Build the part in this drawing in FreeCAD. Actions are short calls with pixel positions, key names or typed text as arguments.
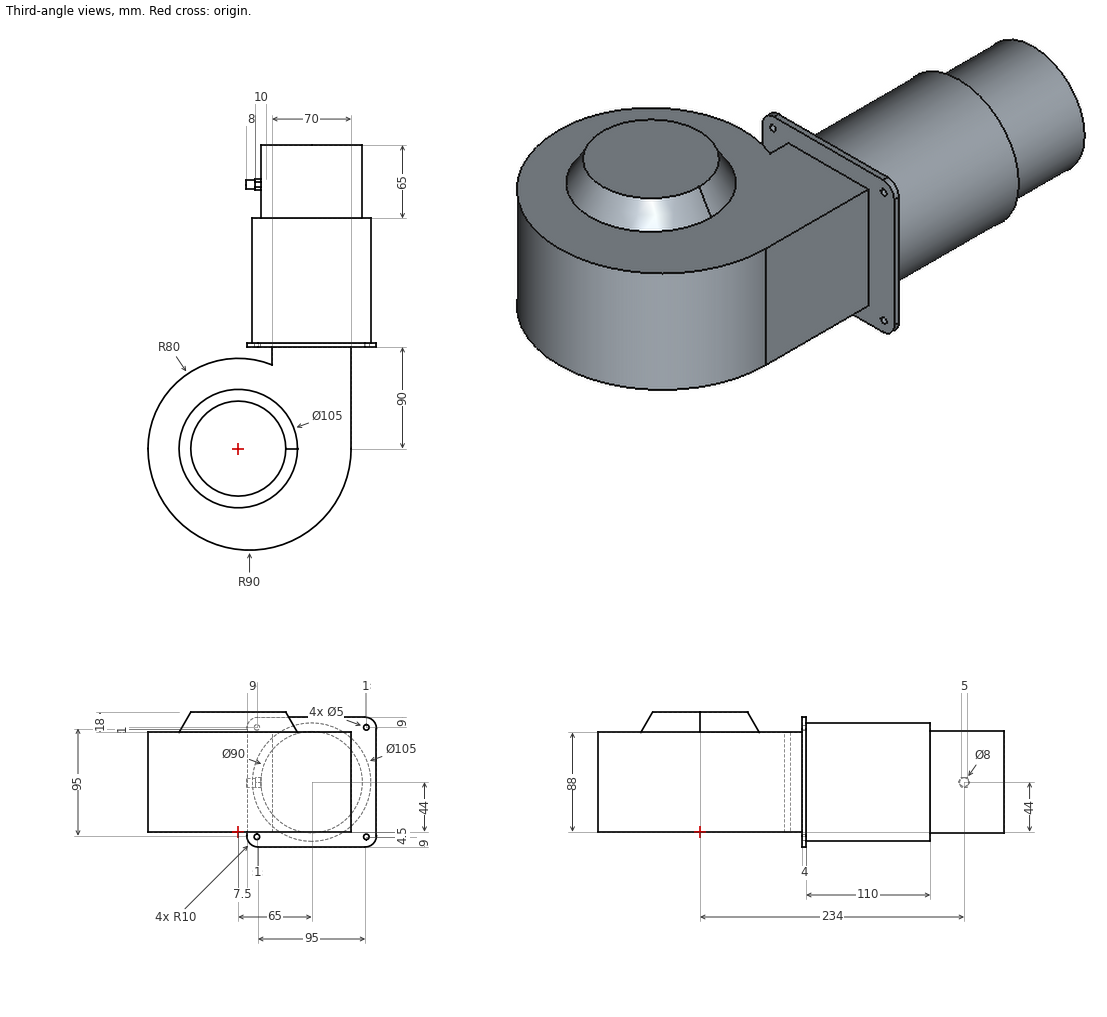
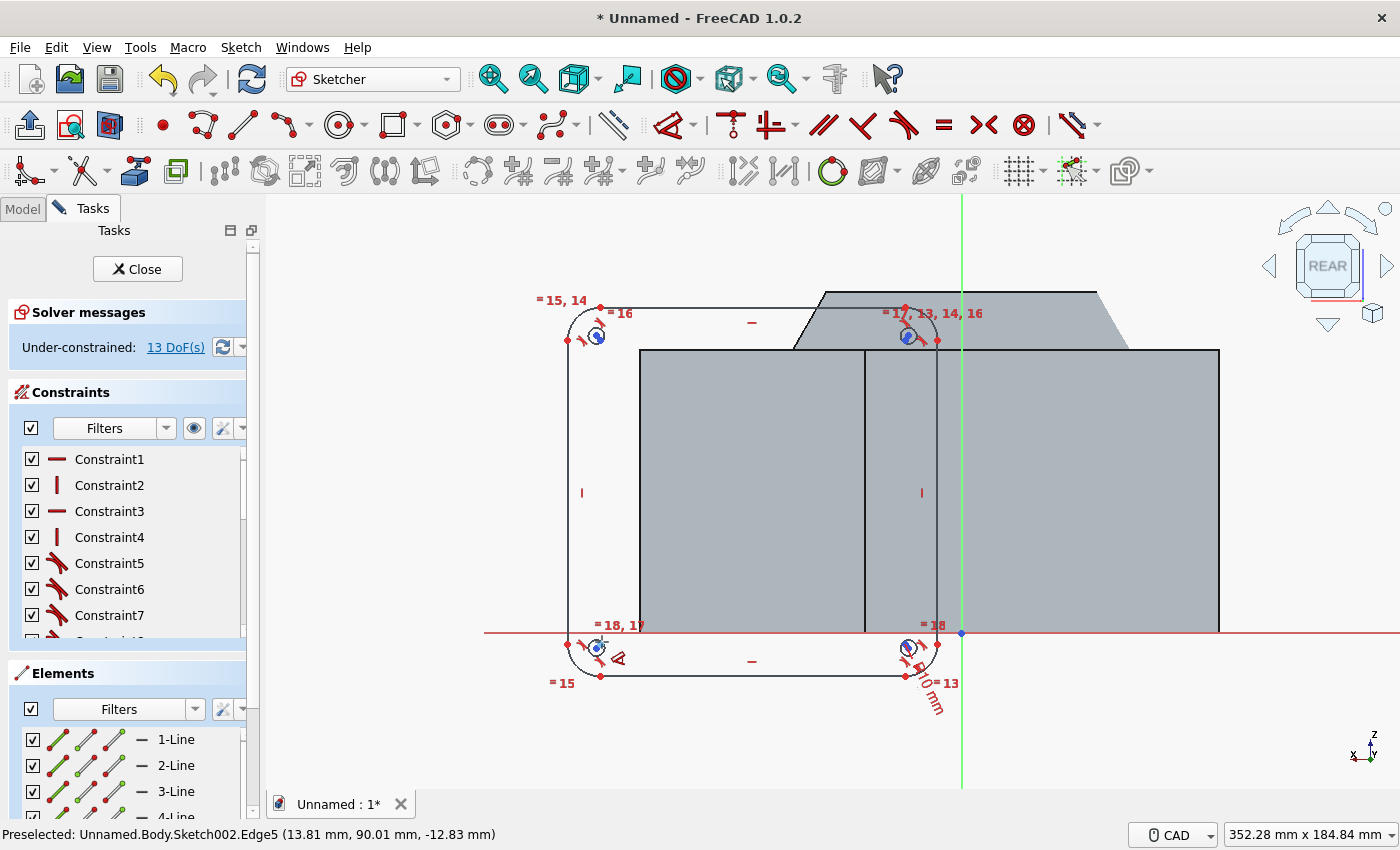
scroll(602, 330, up, 5)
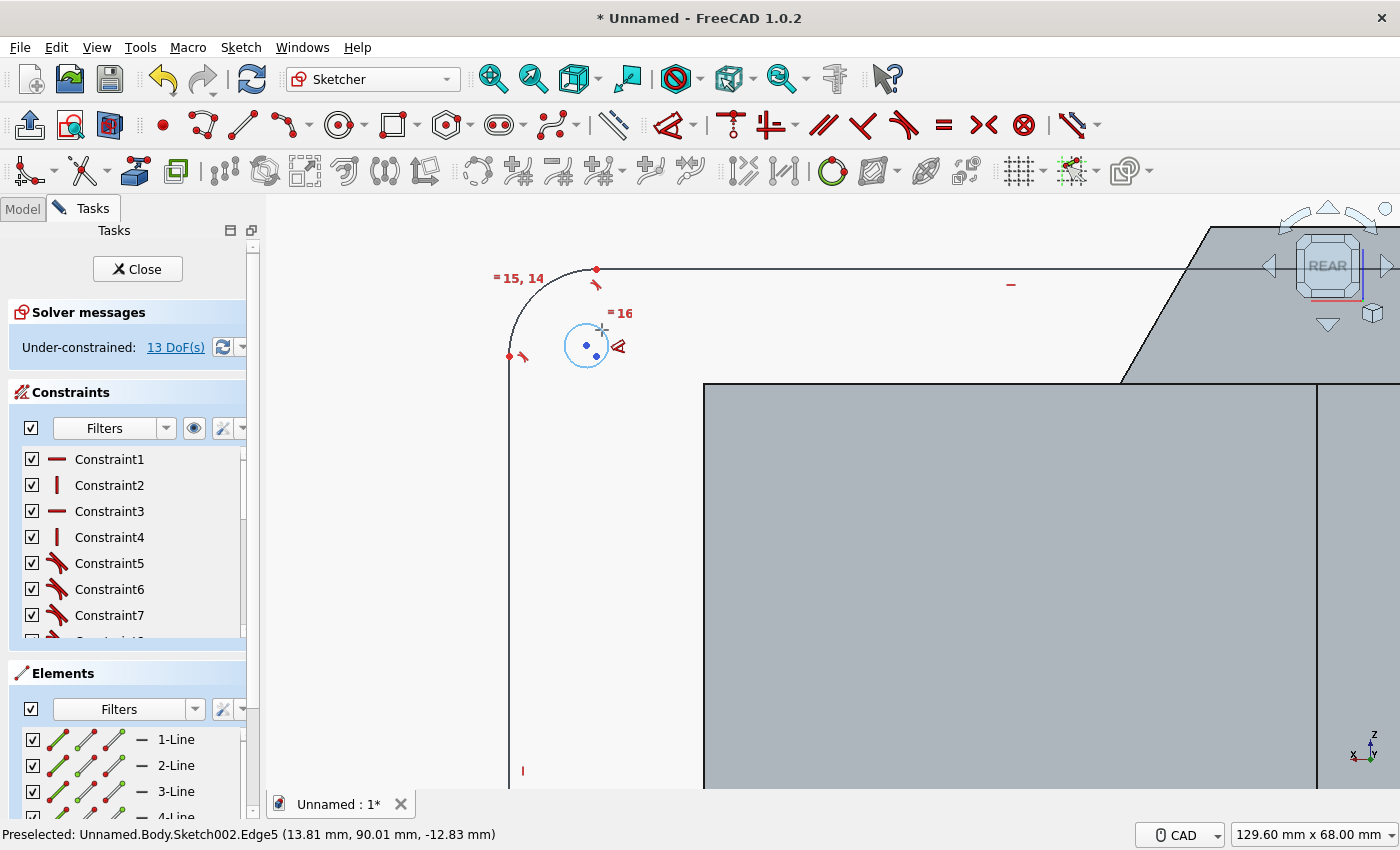
click(602, 330)
click(624, 307)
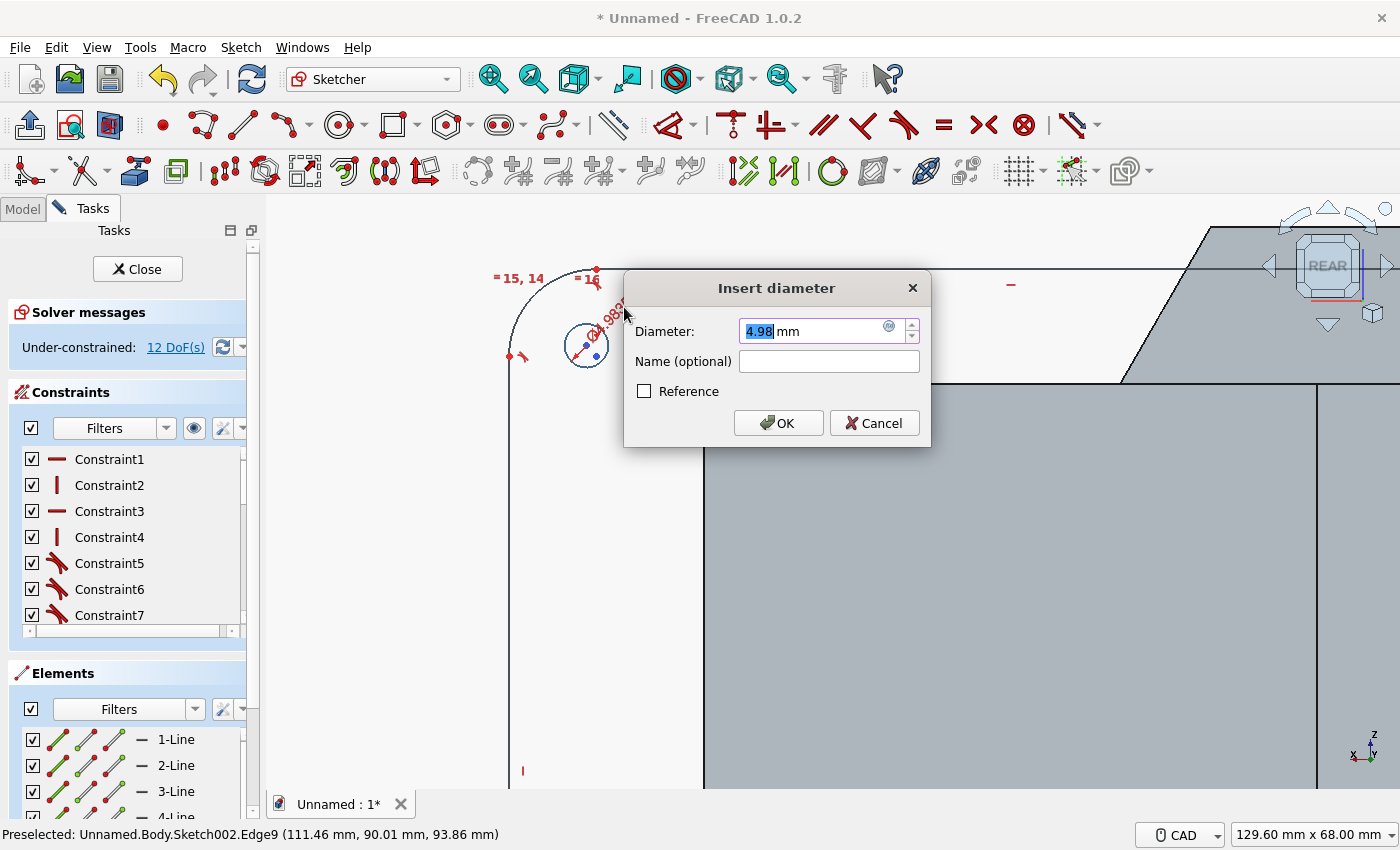
text(5)
key(Return)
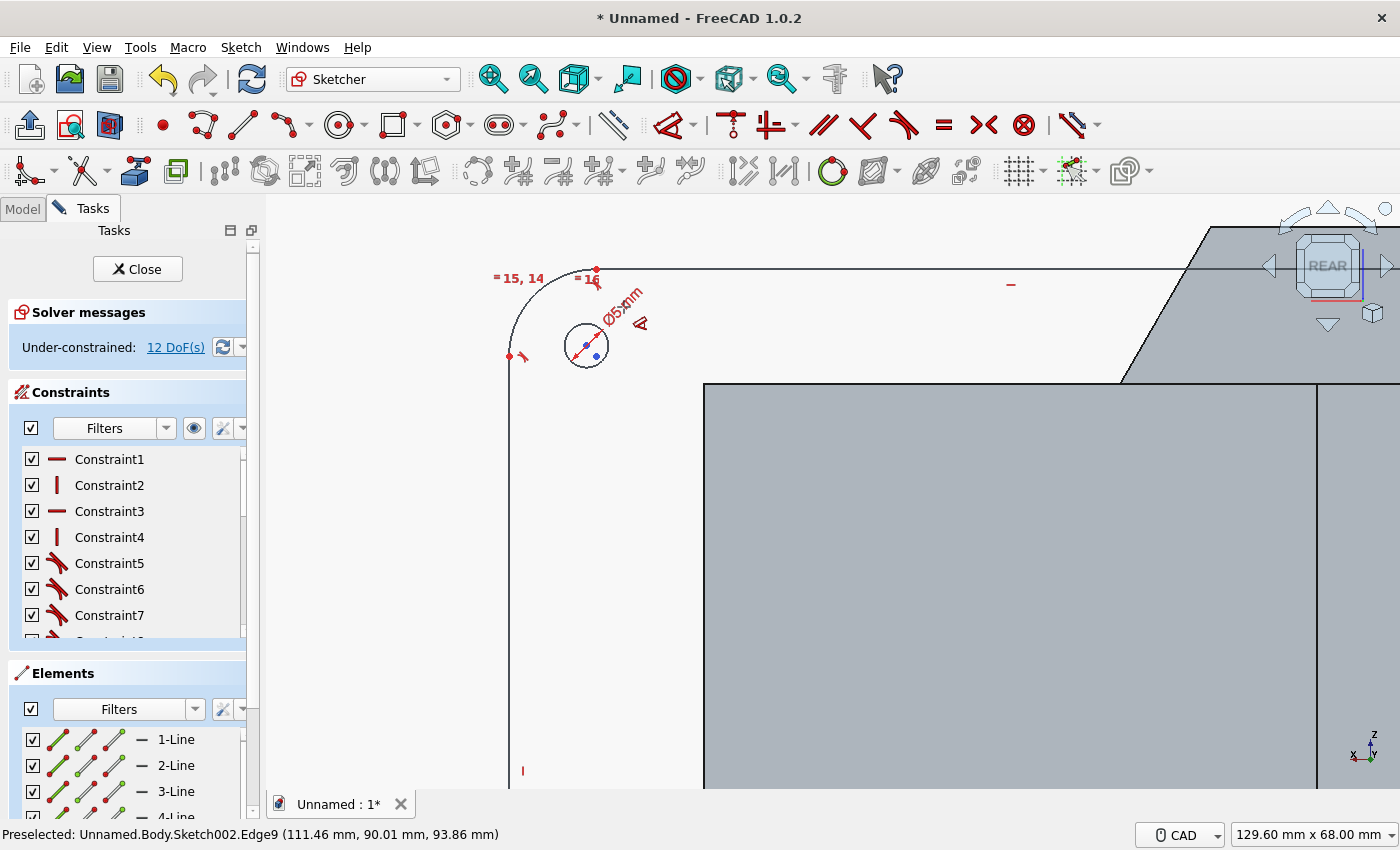
scroll(602, 330, down, 5)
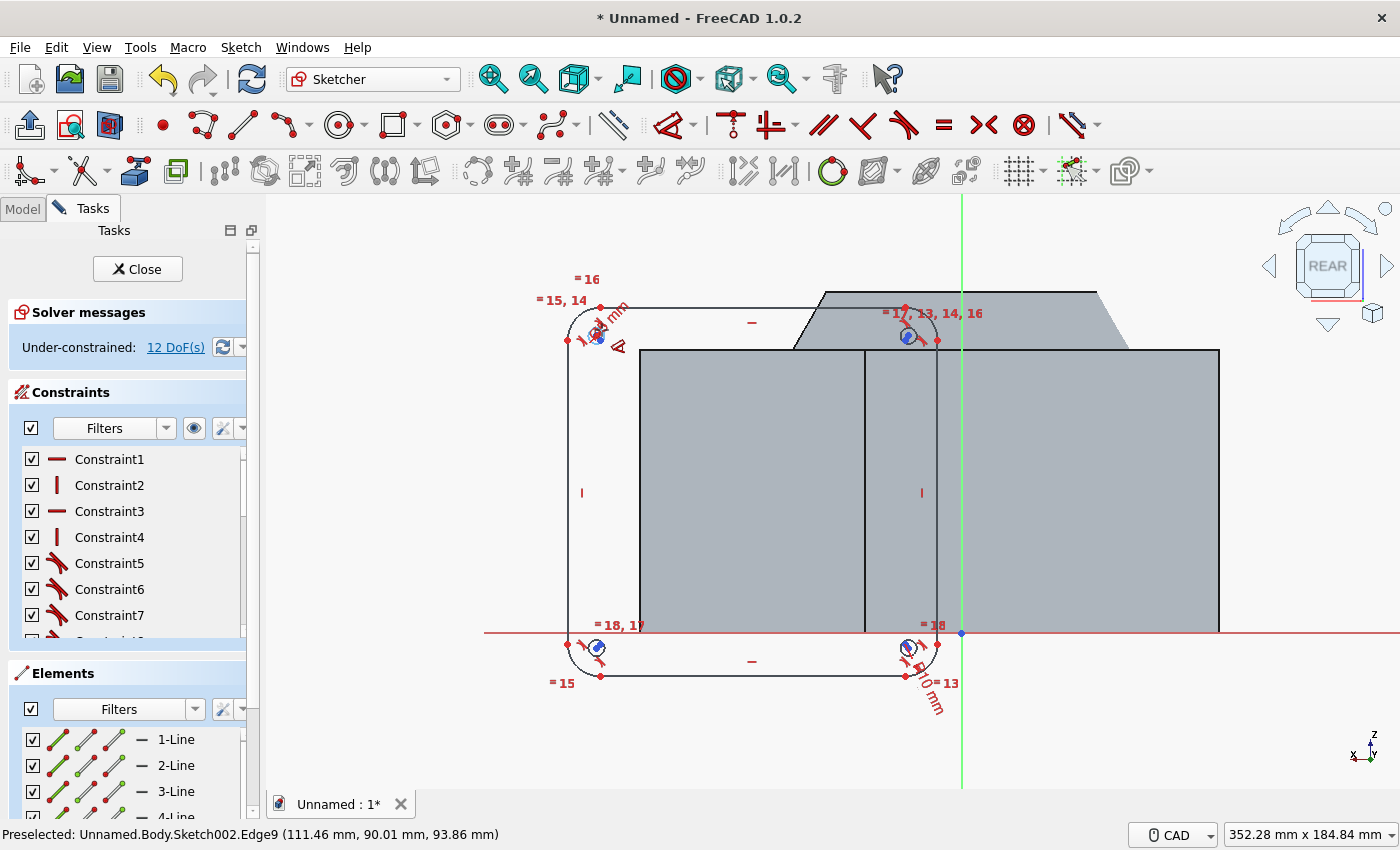
click(692, 676)
click(753, 710)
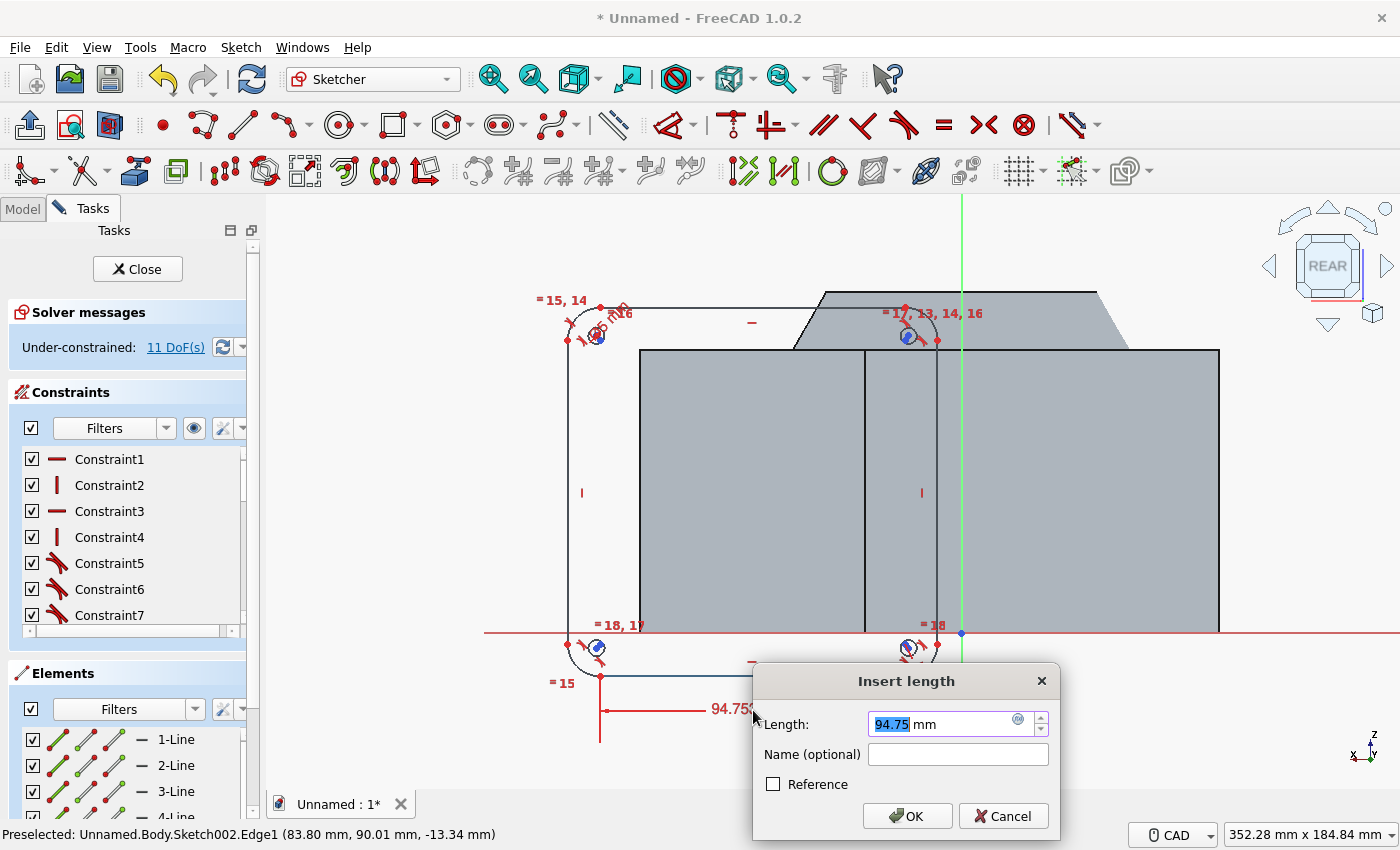
text(95)
key(Return)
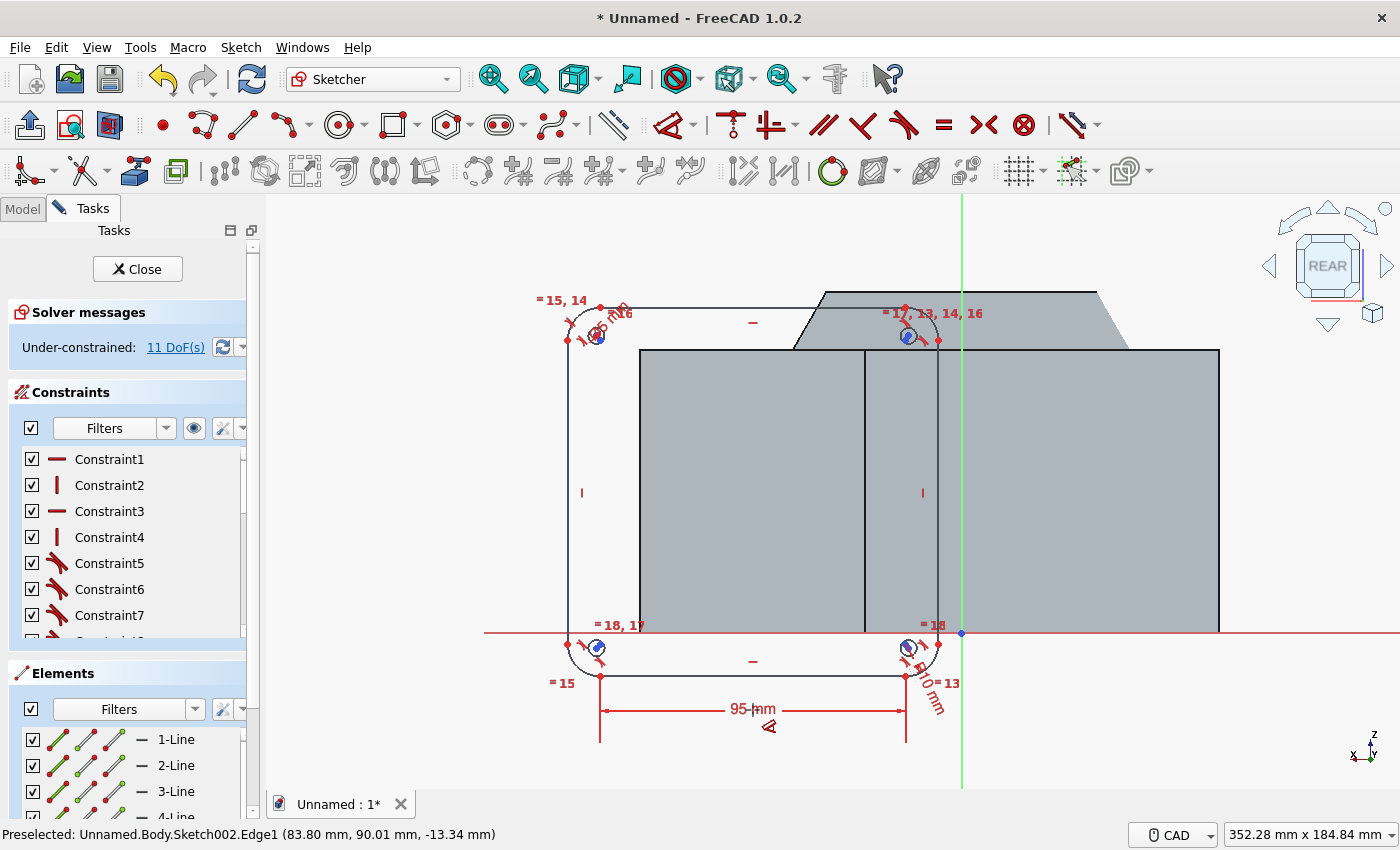
click(938, 553)
click(904, 492)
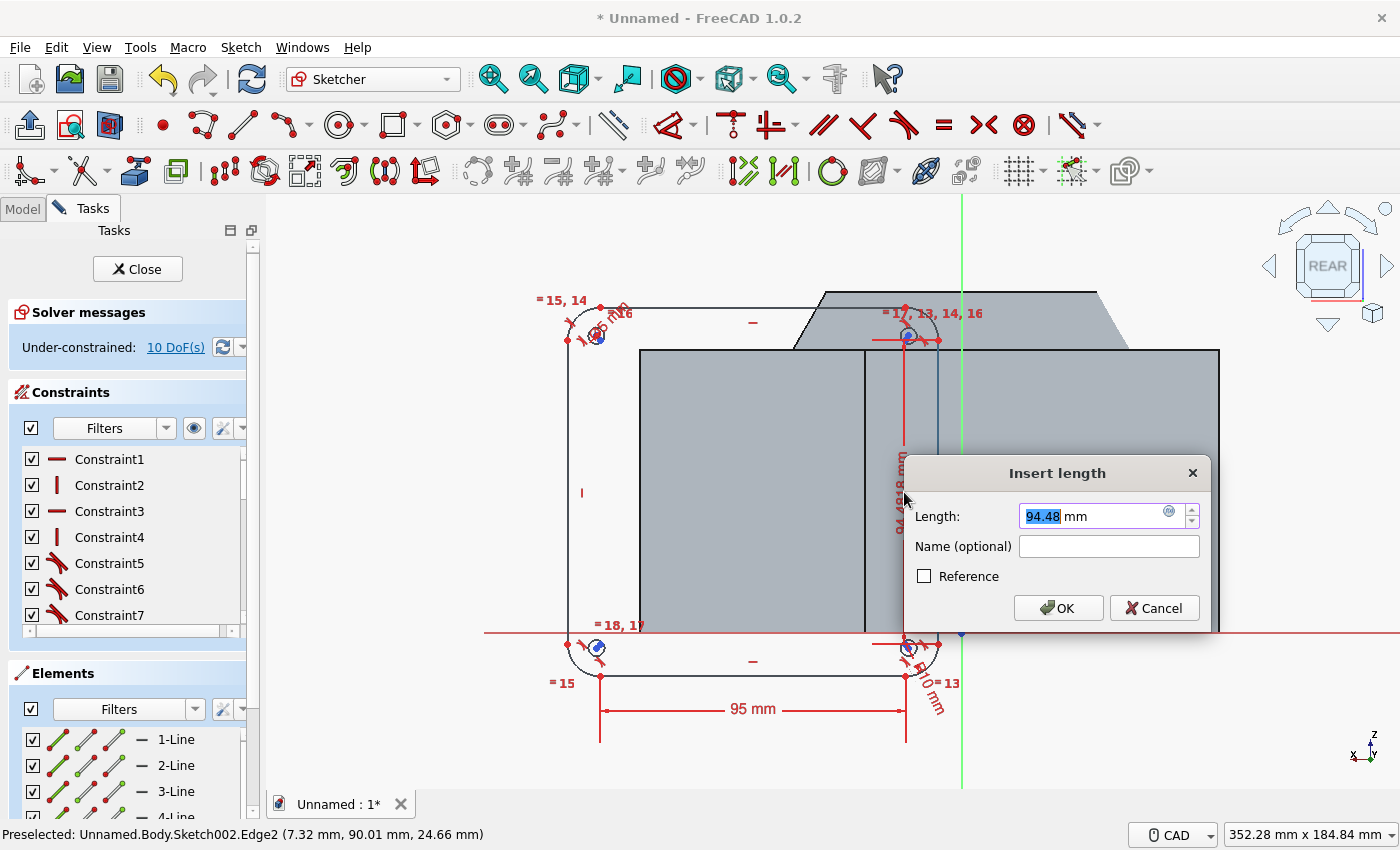
text(95)
key(Return)